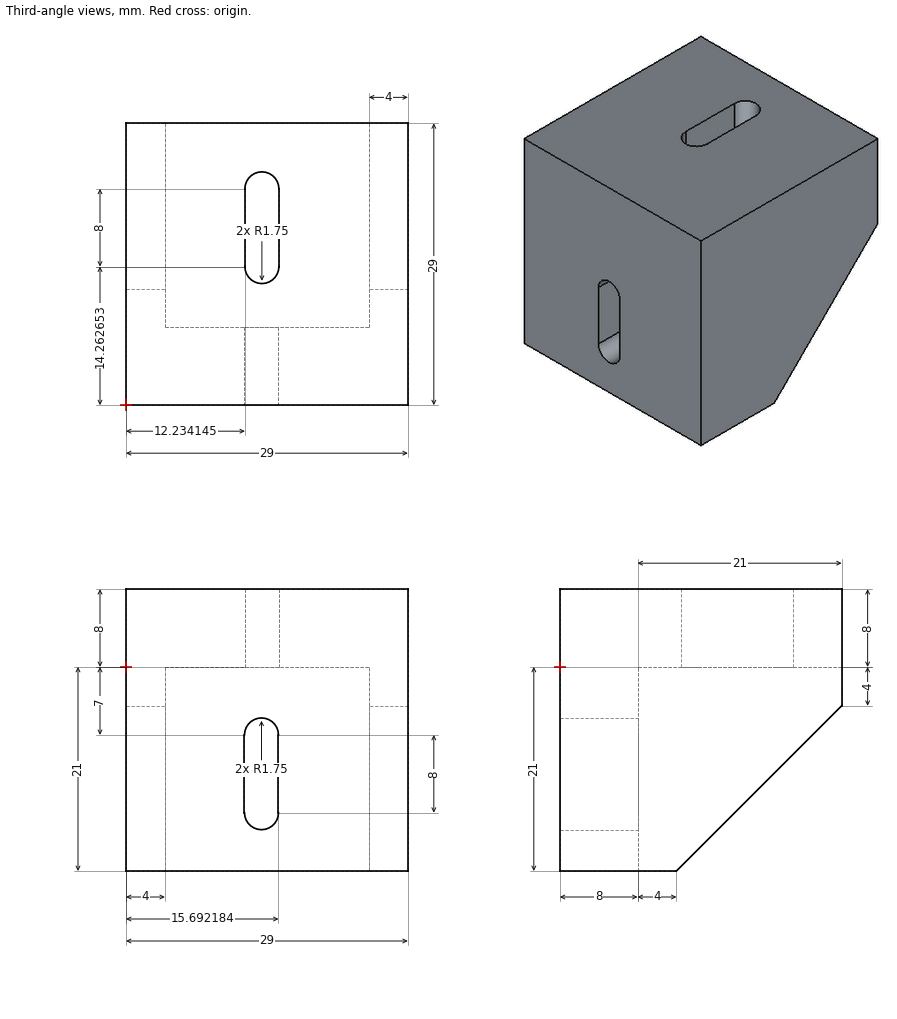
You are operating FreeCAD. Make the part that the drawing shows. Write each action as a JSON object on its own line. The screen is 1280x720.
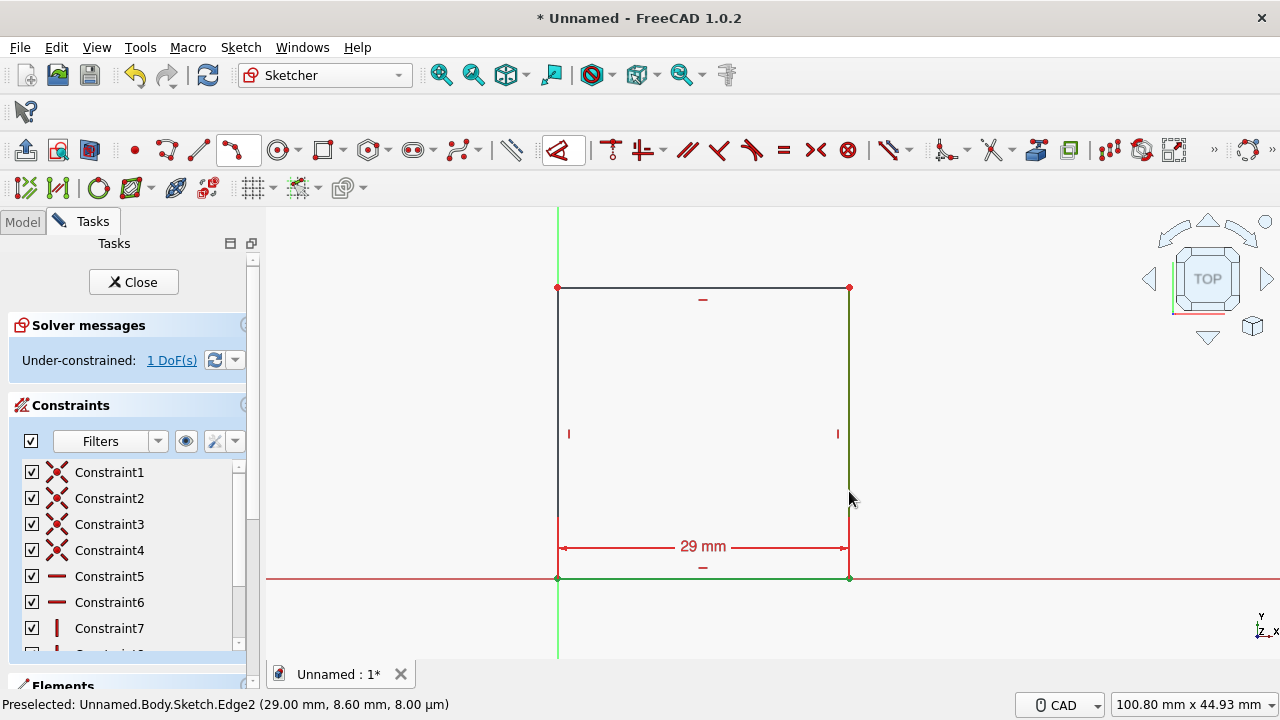
{"action": "key", "text": "i"}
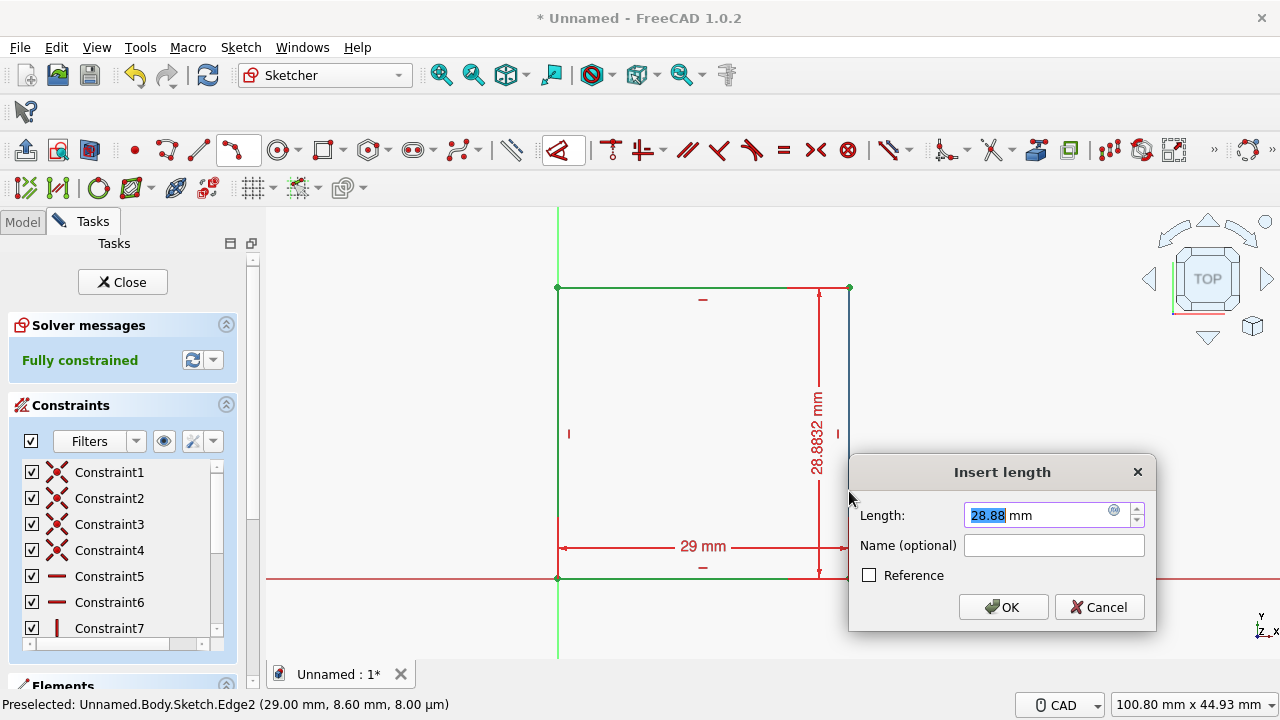
{"action": "type", "text": "29"}
{"action": "key", "text": "Return"}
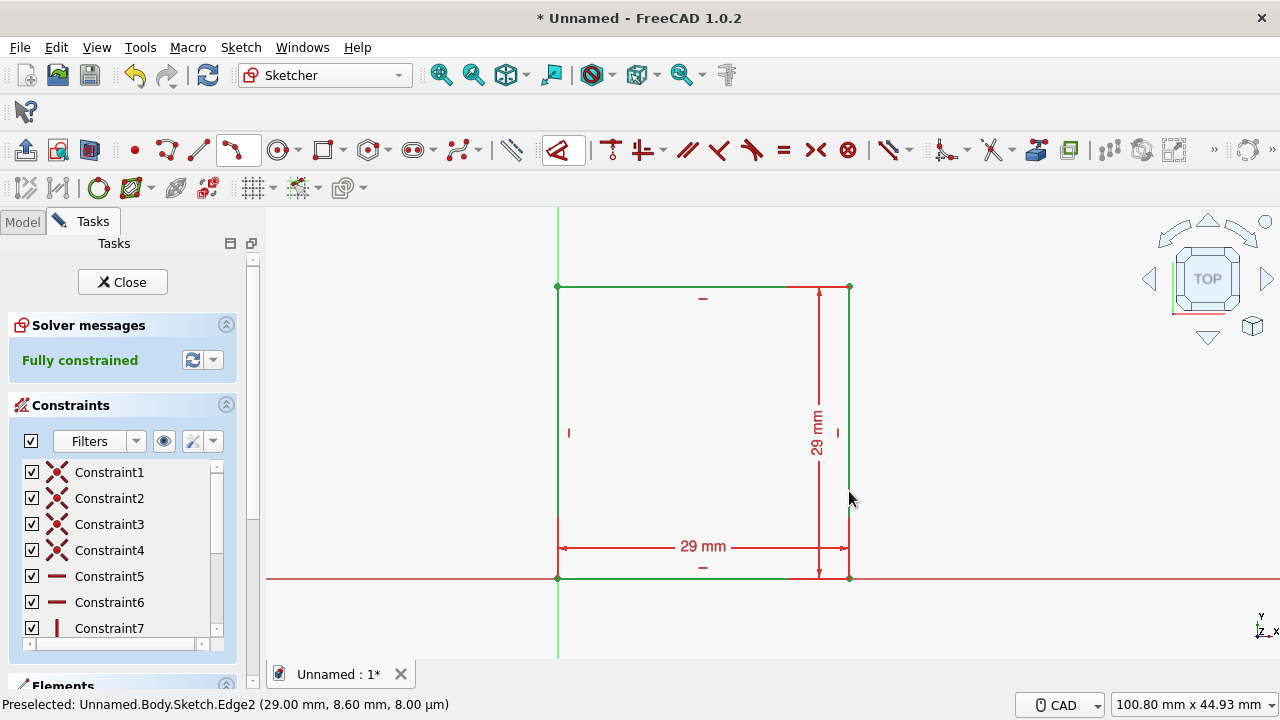
{"action": "left_click", "coordinate": [123, 282]}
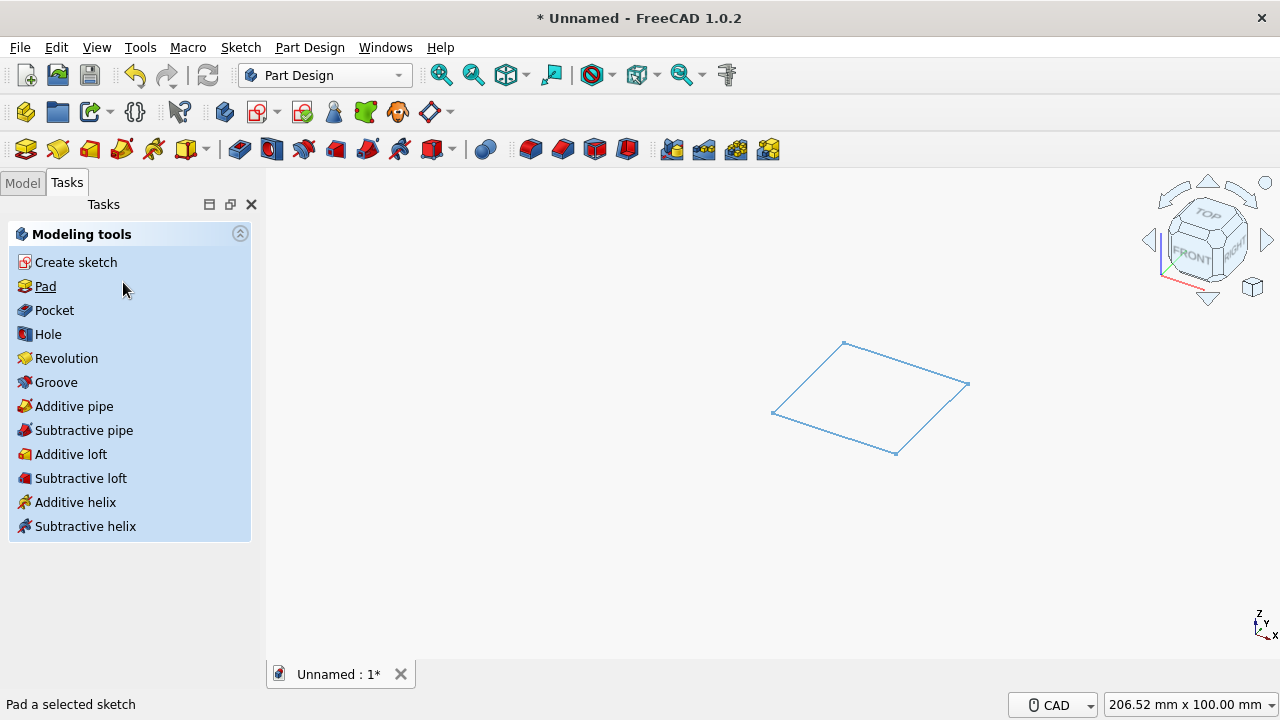
{"action": "left_click", "coordinate": [26, 150]}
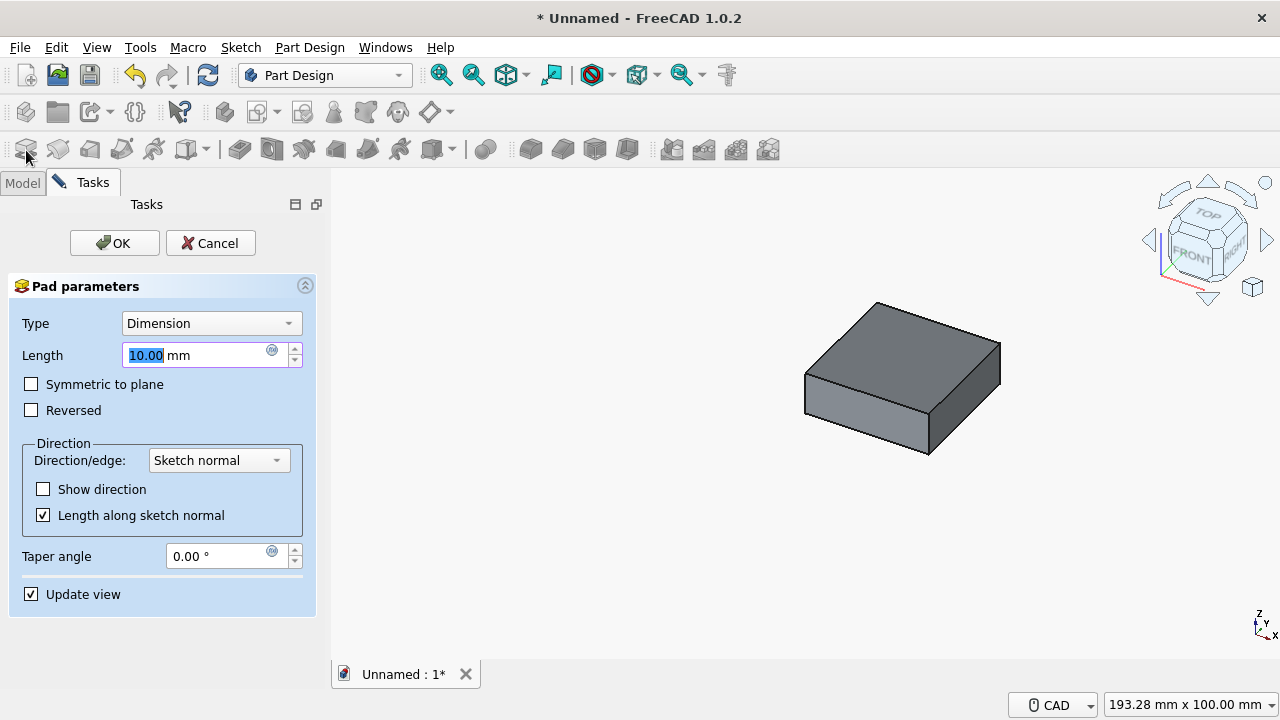
{"action": "type", "text": "8"}
{"action": "key", "text": "Tab"}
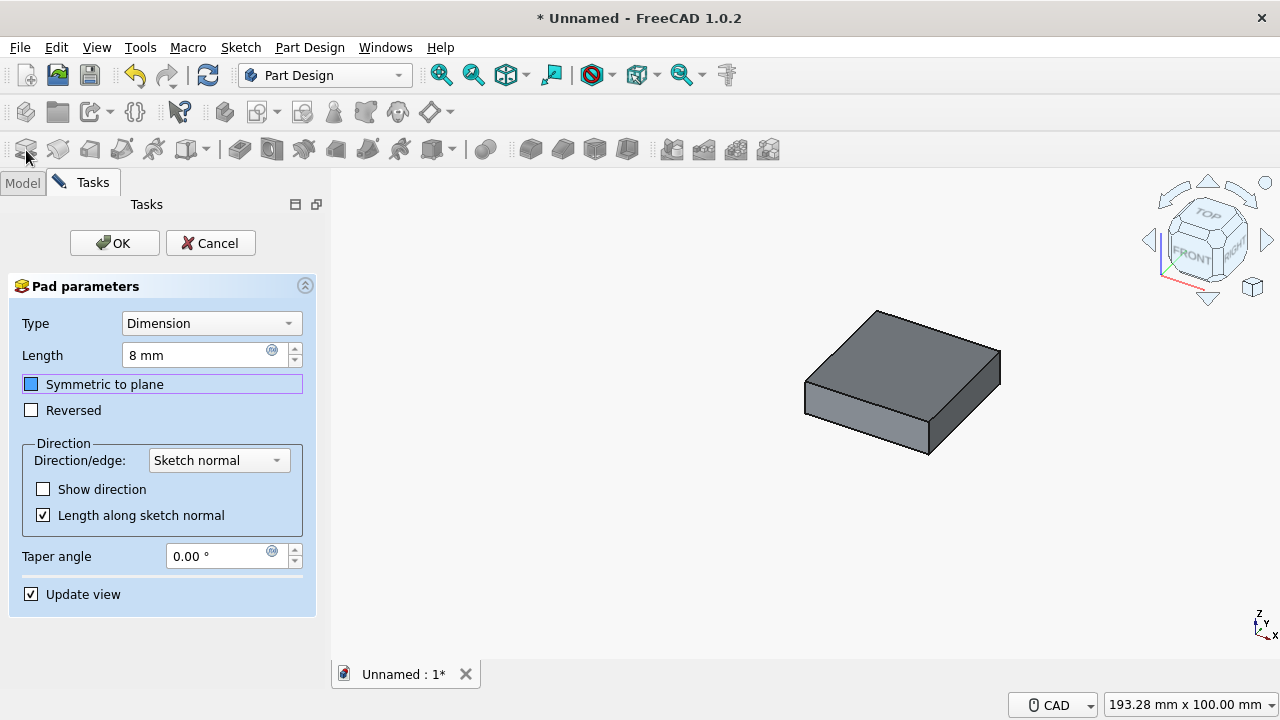
{"action": "left_click", "coordinate": [115, 243]}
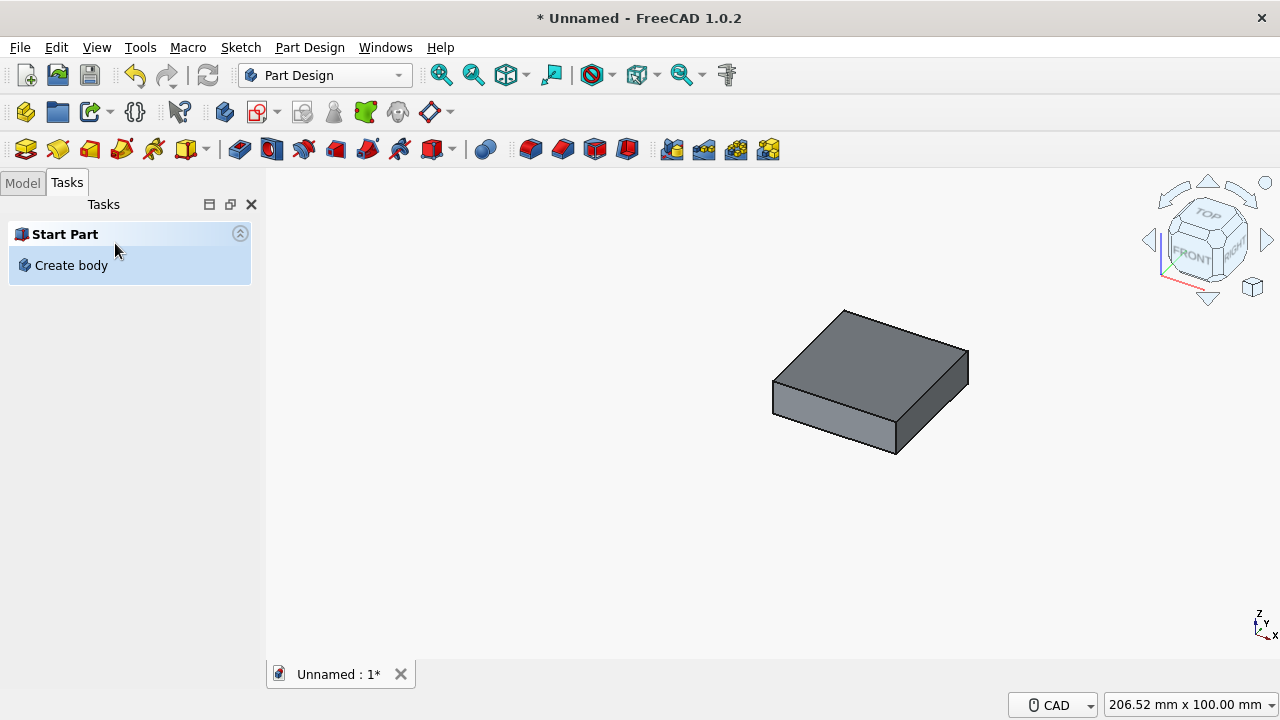
{"action": "left_click", "coordinate": [442, 76]}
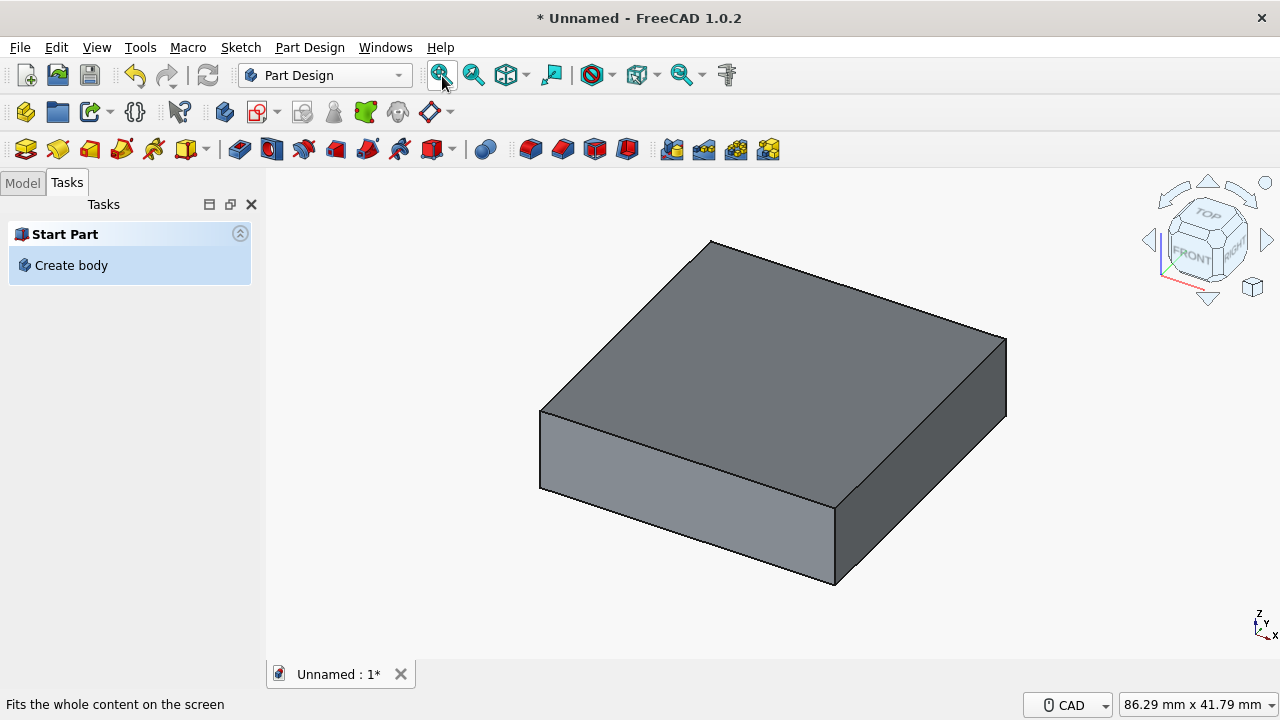
{"action": "left_click", "coordinate": [773, 374]}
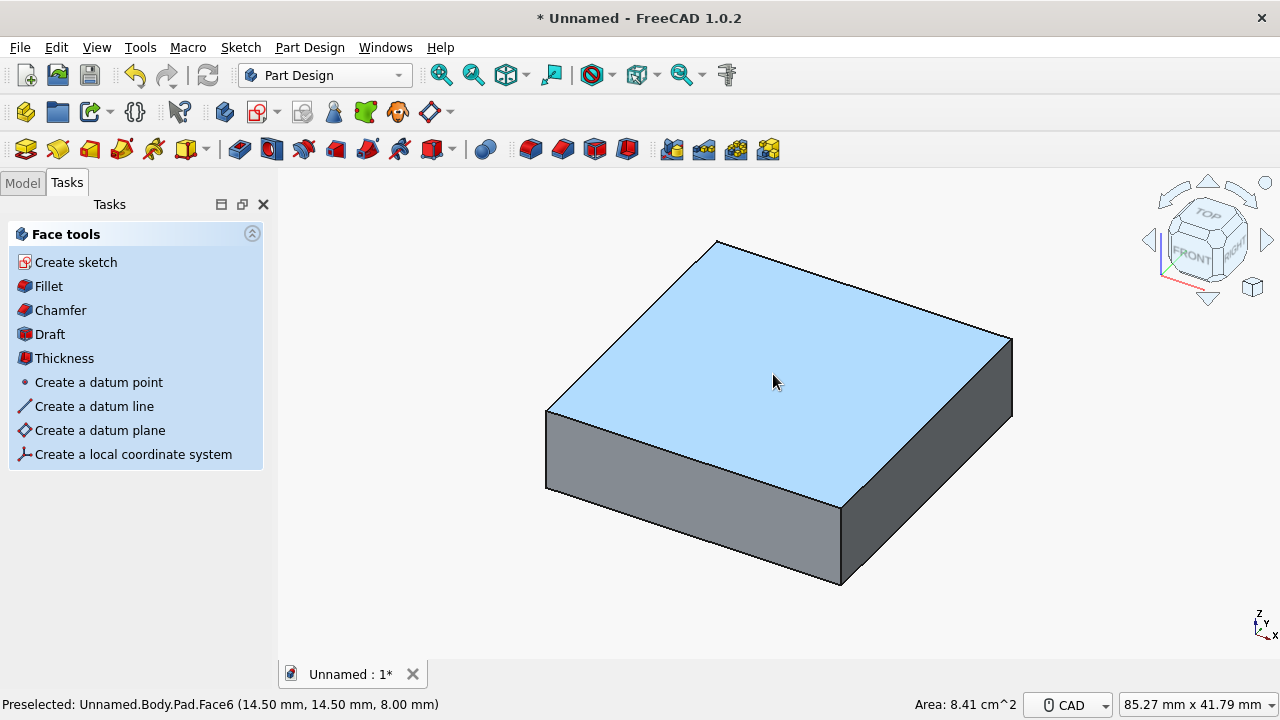
{"action": "left_click", "coordinate": [258, 112]}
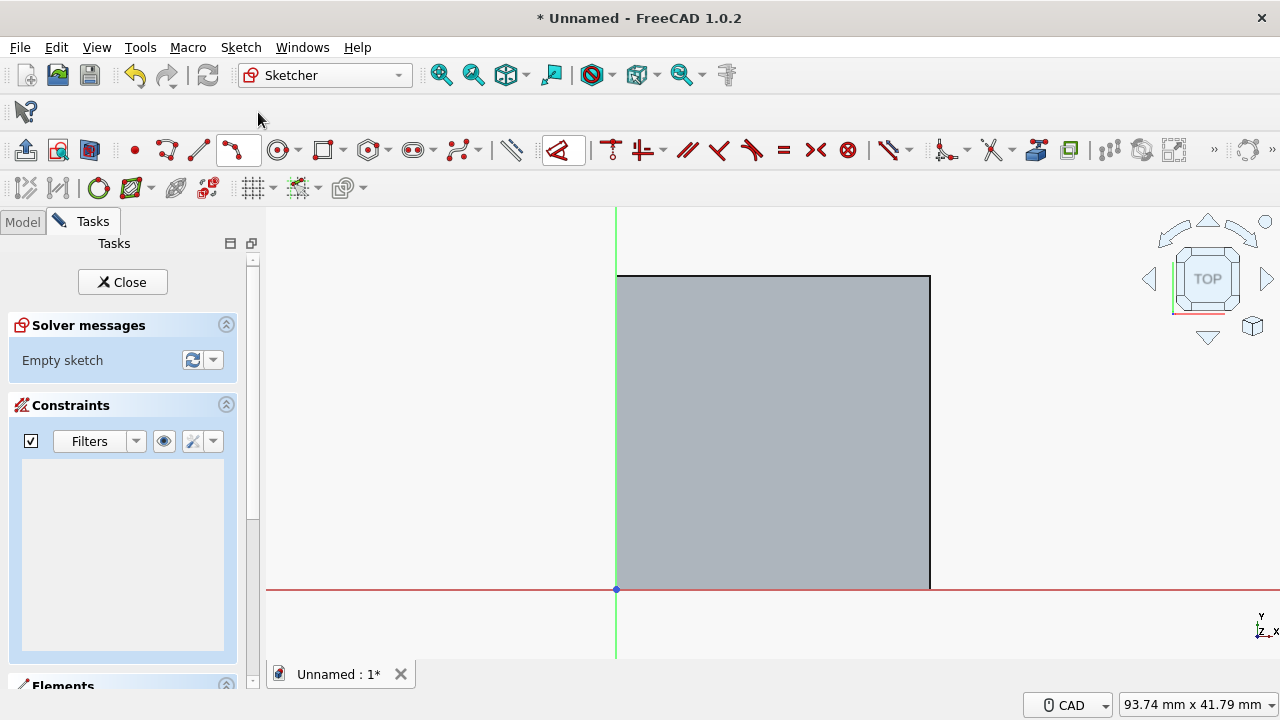
{"action": "left_click", "coordinate": [414, 150]}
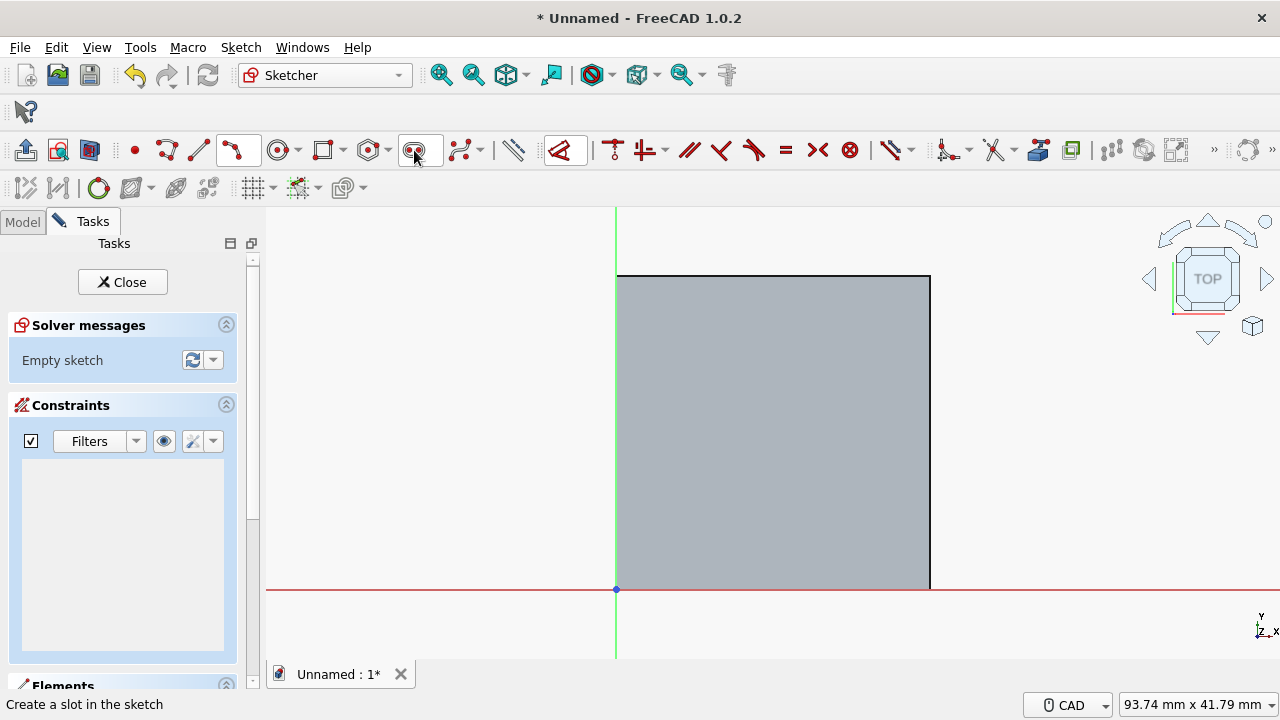
{"action": "left_click", "coordinate": [767, 436]}